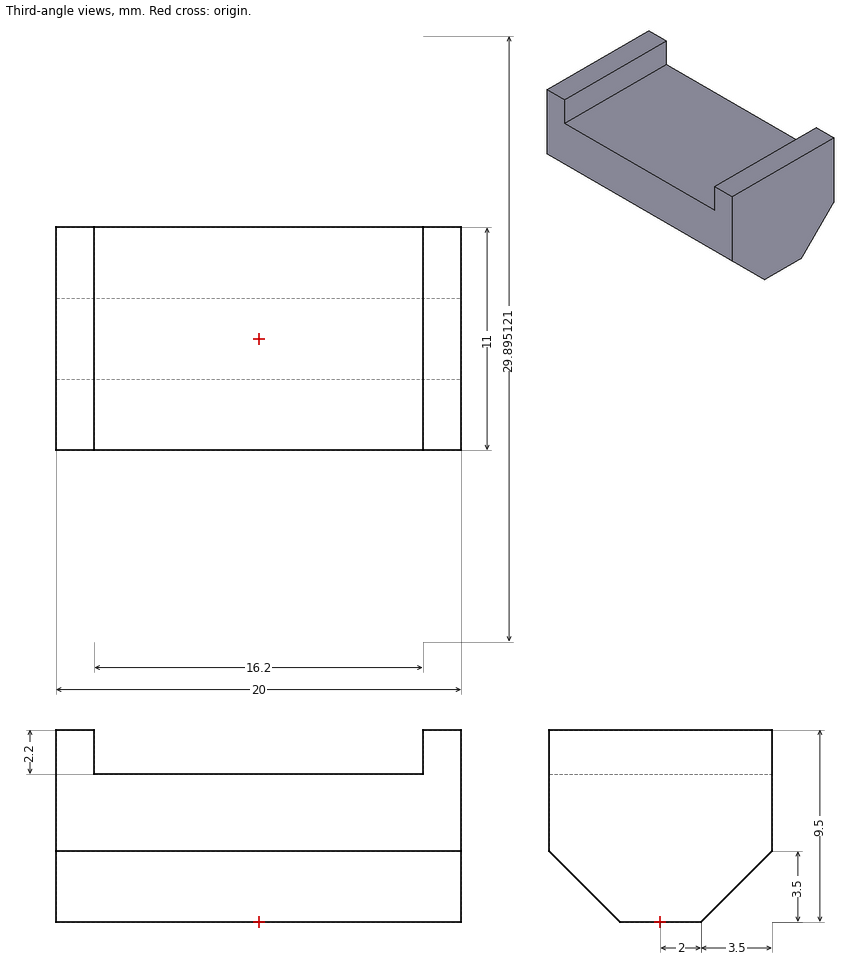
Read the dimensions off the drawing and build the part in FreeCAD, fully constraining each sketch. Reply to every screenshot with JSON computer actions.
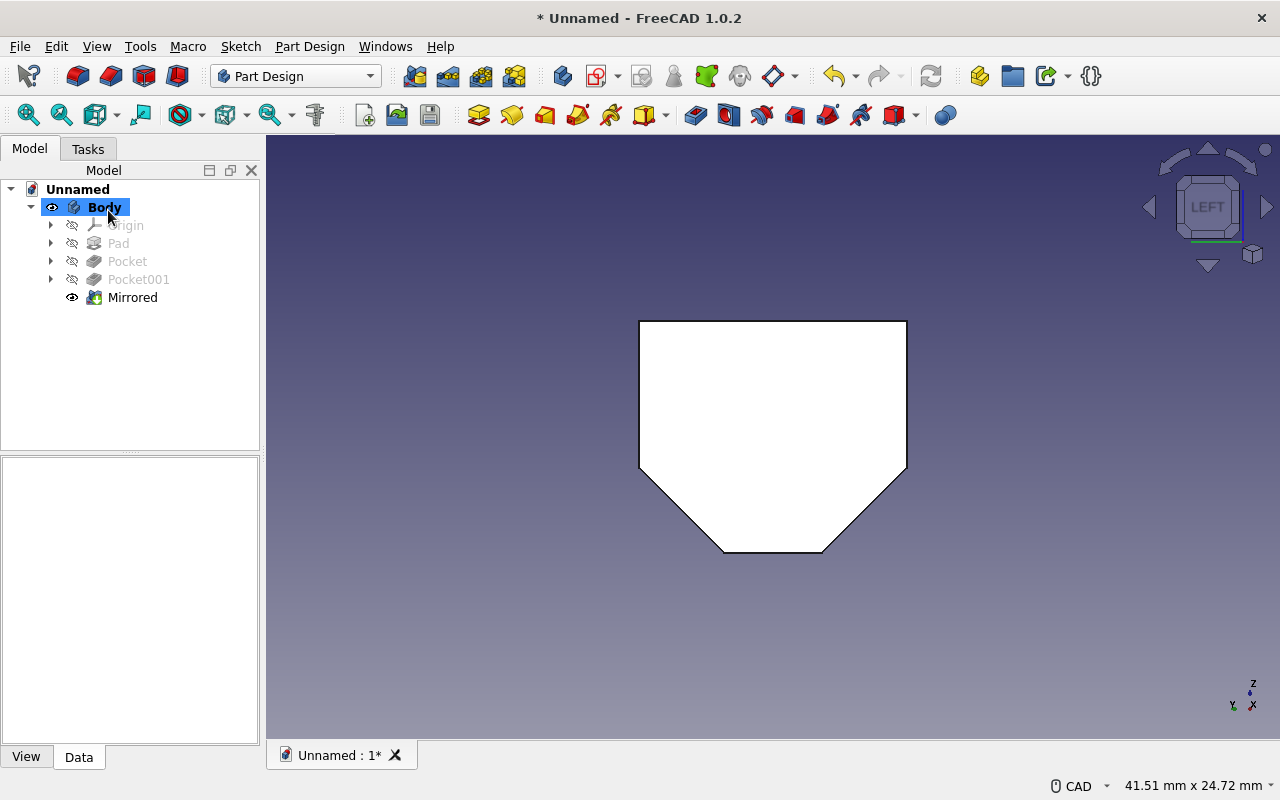
{"action": "key", "text": "0"}